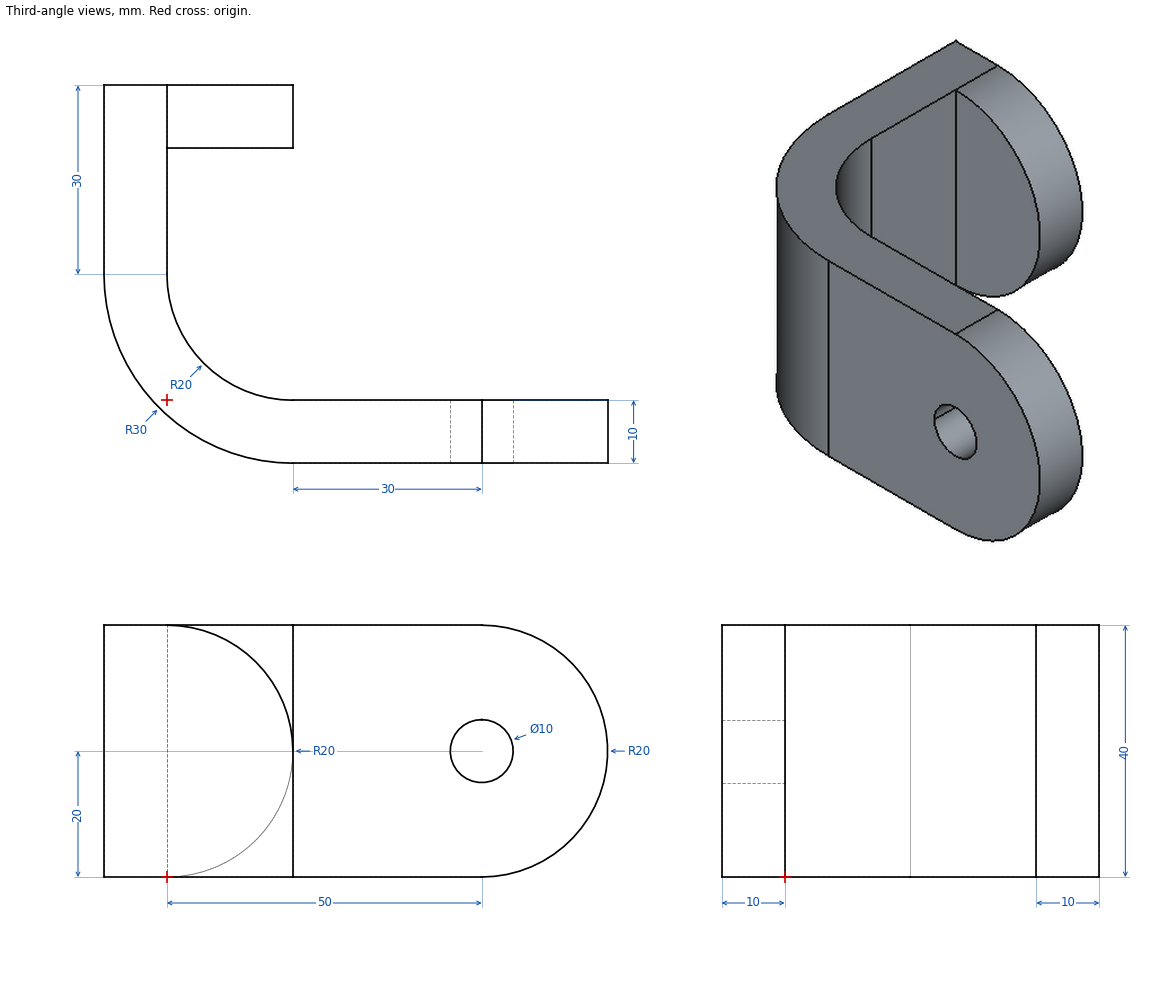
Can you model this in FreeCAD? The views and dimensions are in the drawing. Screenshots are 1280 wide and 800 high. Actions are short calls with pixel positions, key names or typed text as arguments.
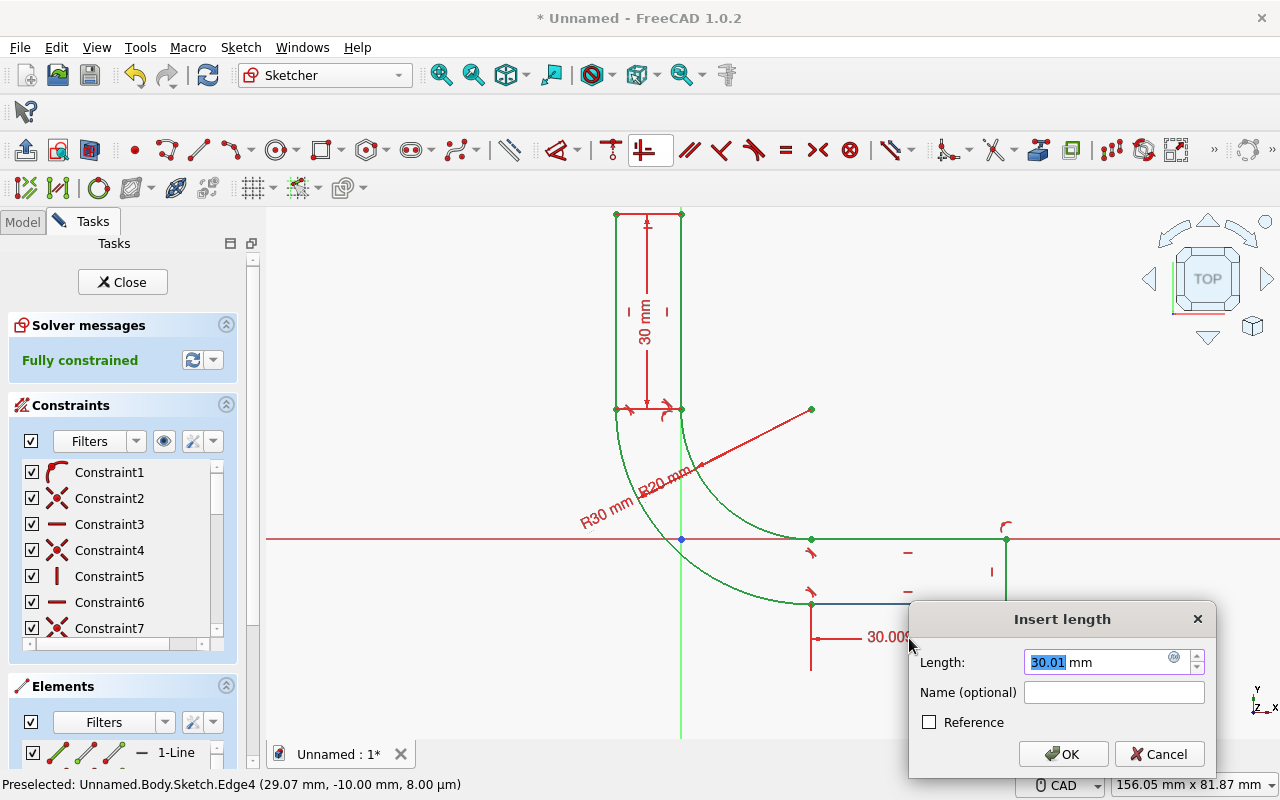
text(30)
key(Return)
key(Escape)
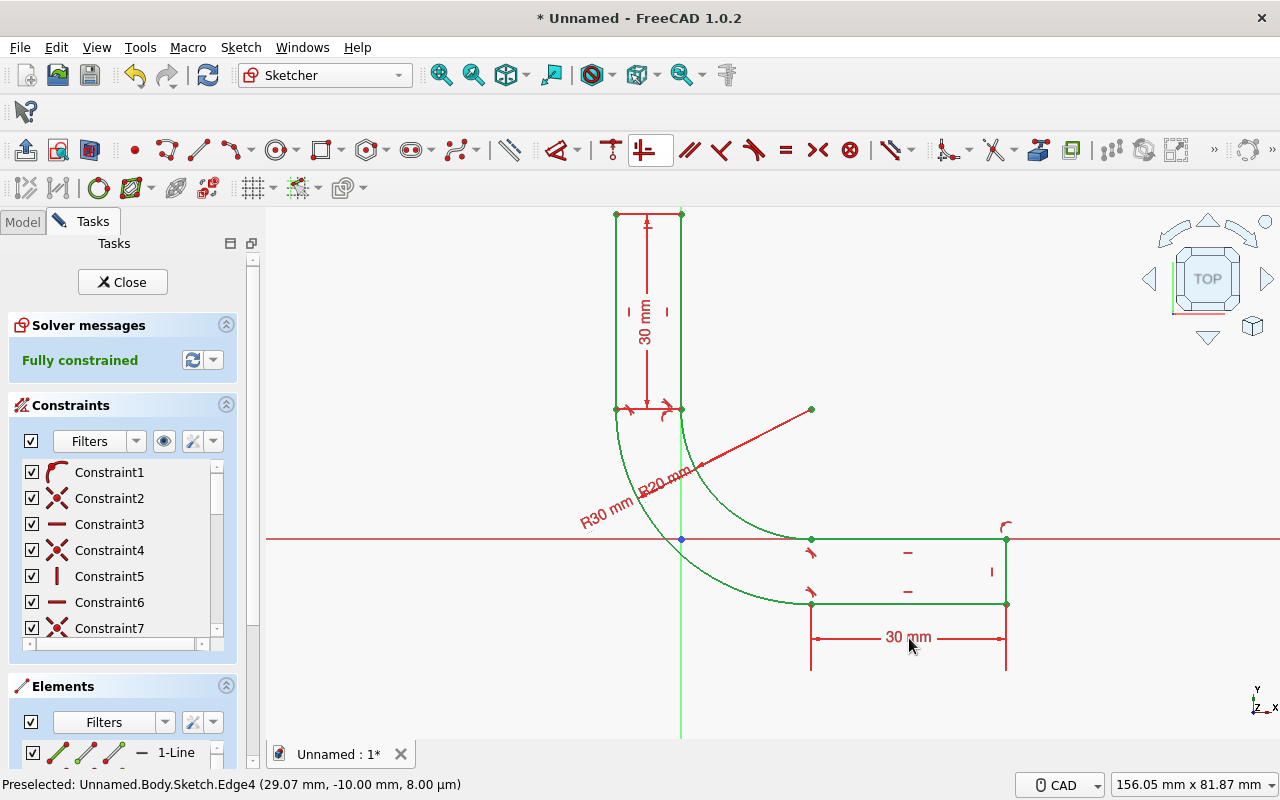
click(123, 282)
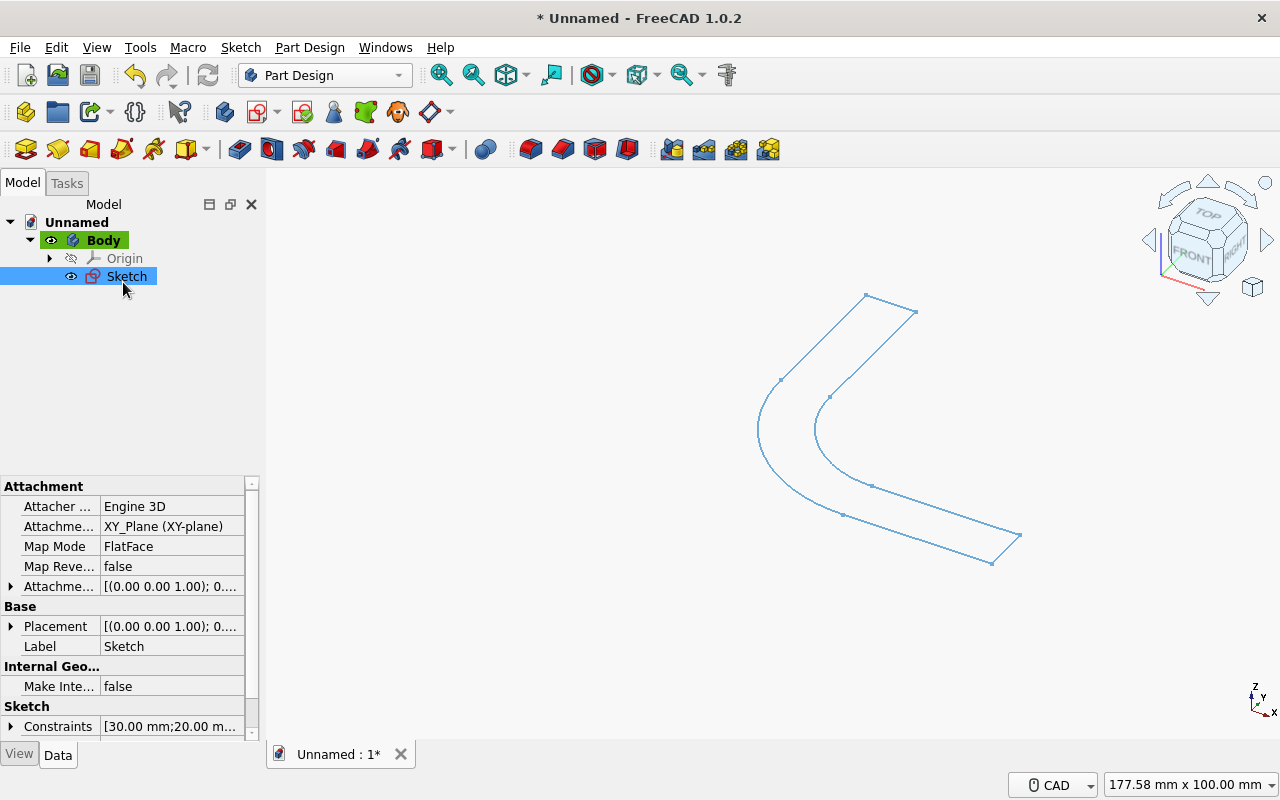
click(26, 150)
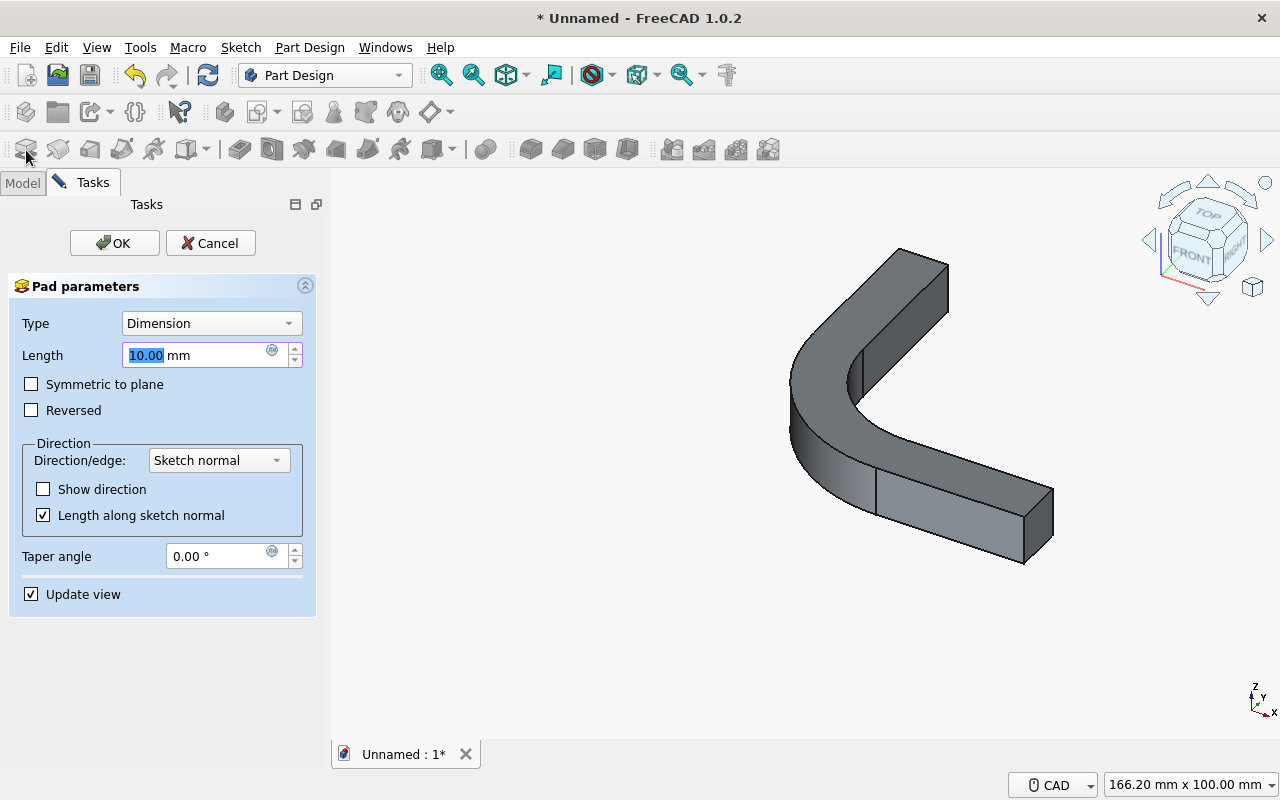
text(40)
key(Tab)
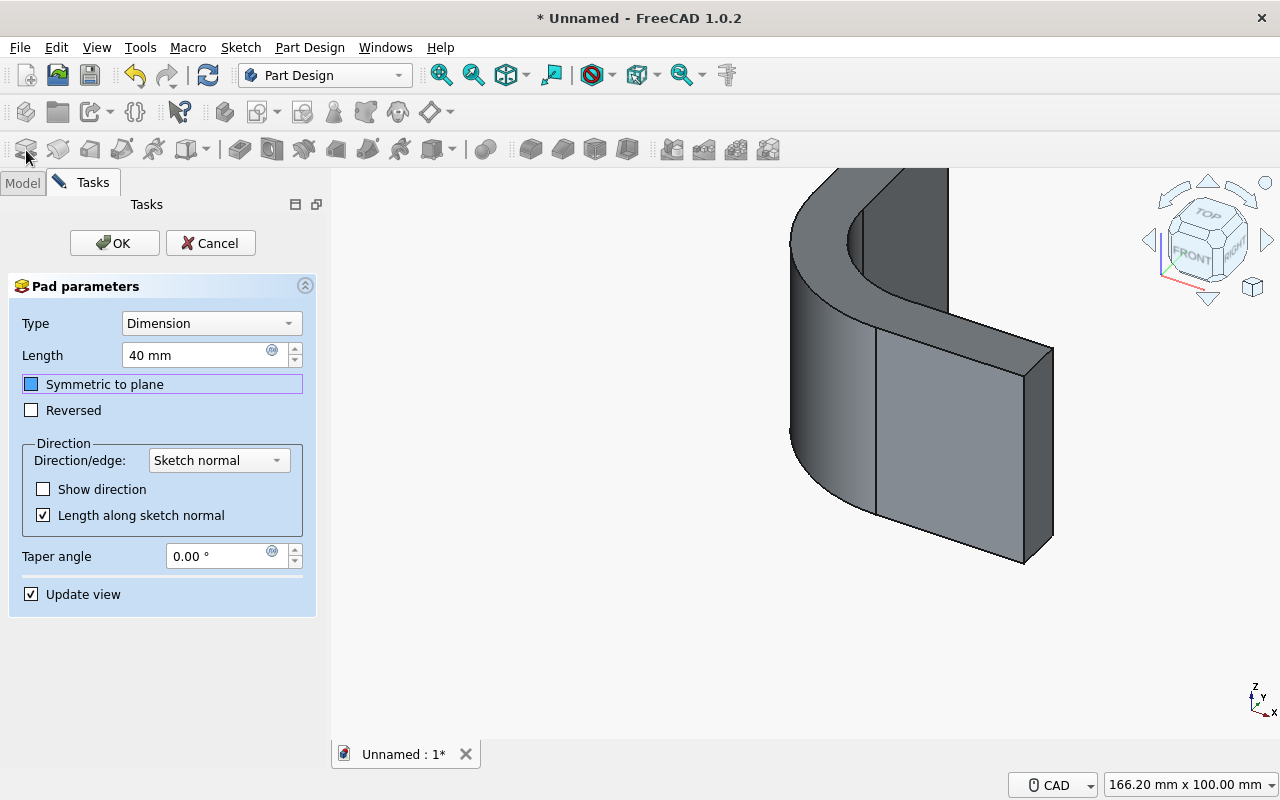
click(115, 243)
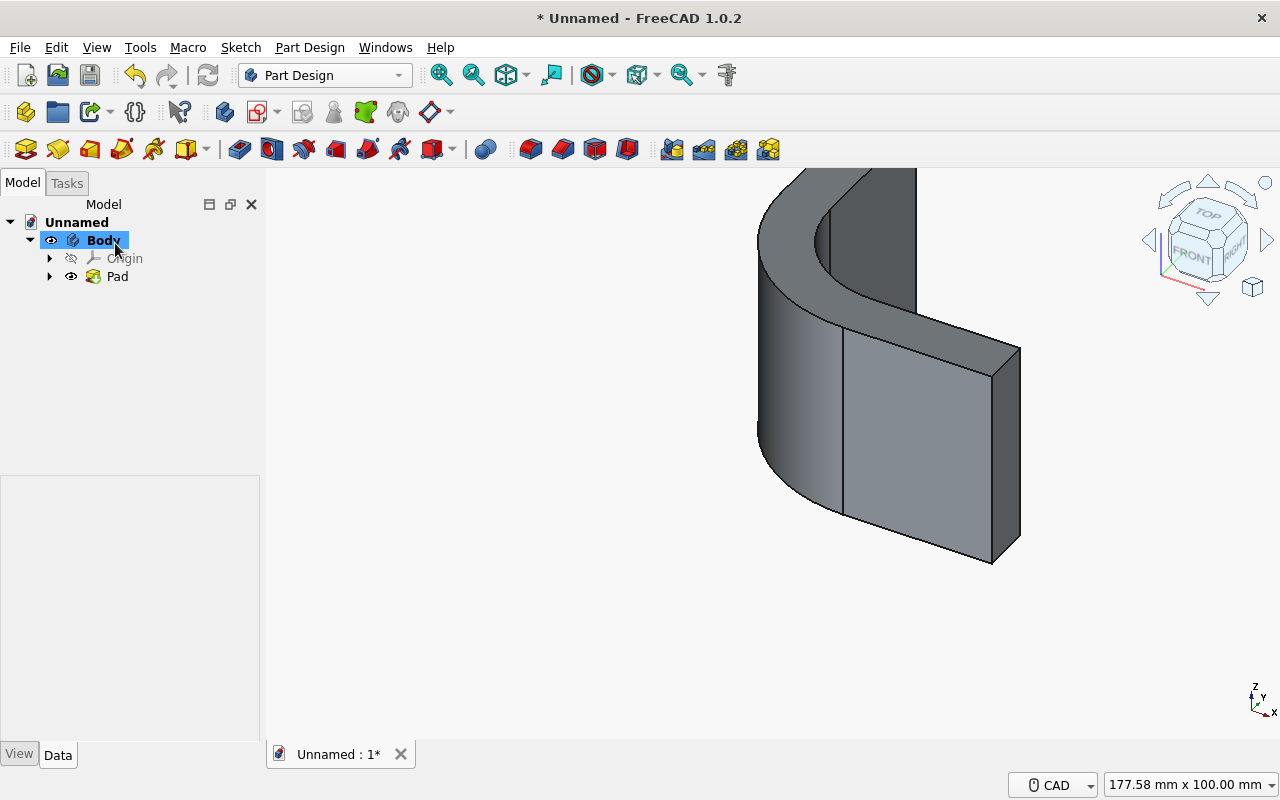
key(v)
key(f)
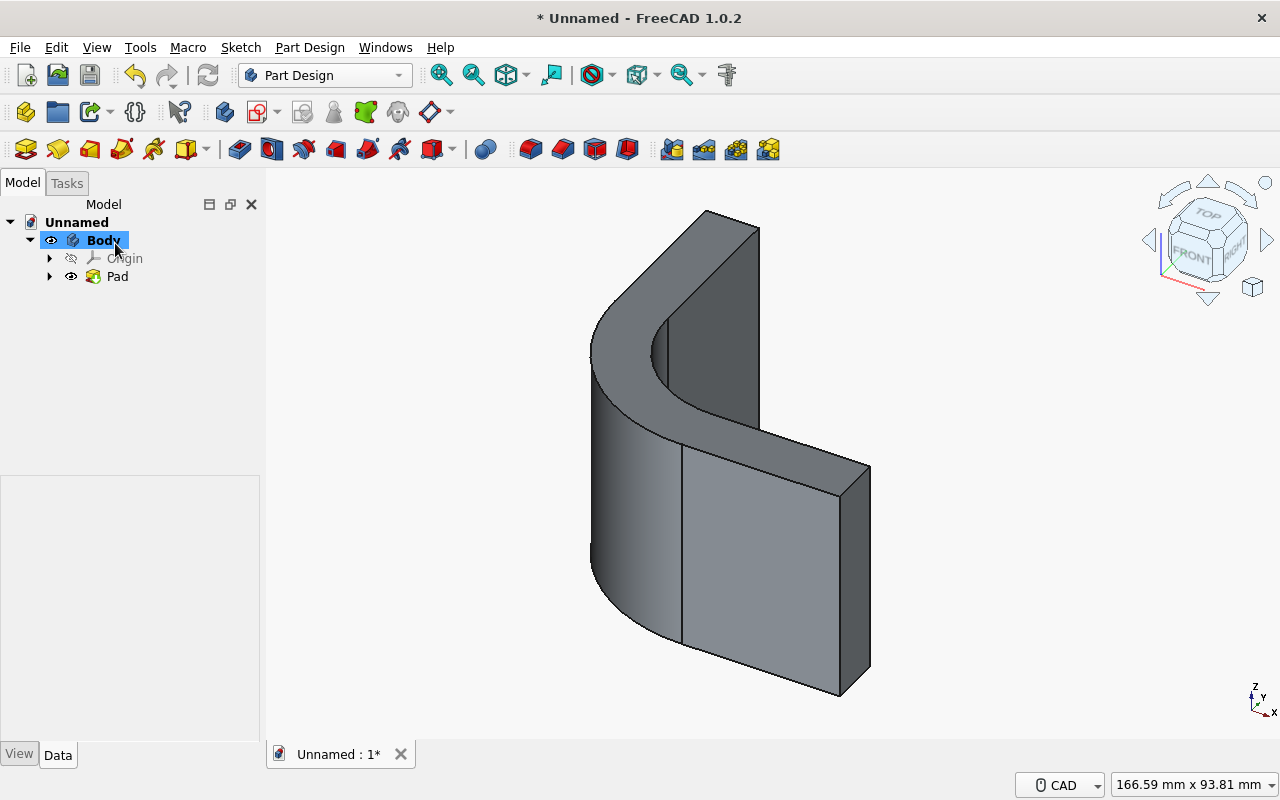
key(4)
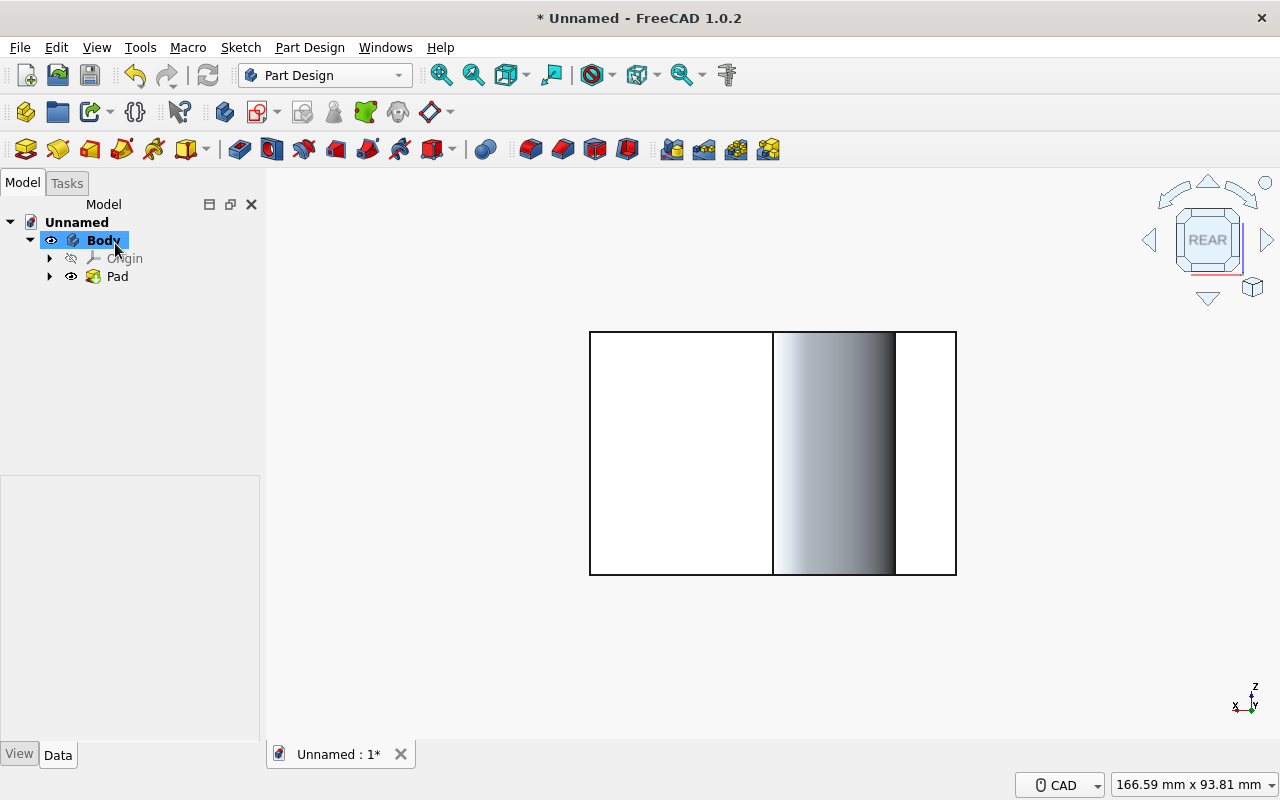
key(v)
key(f)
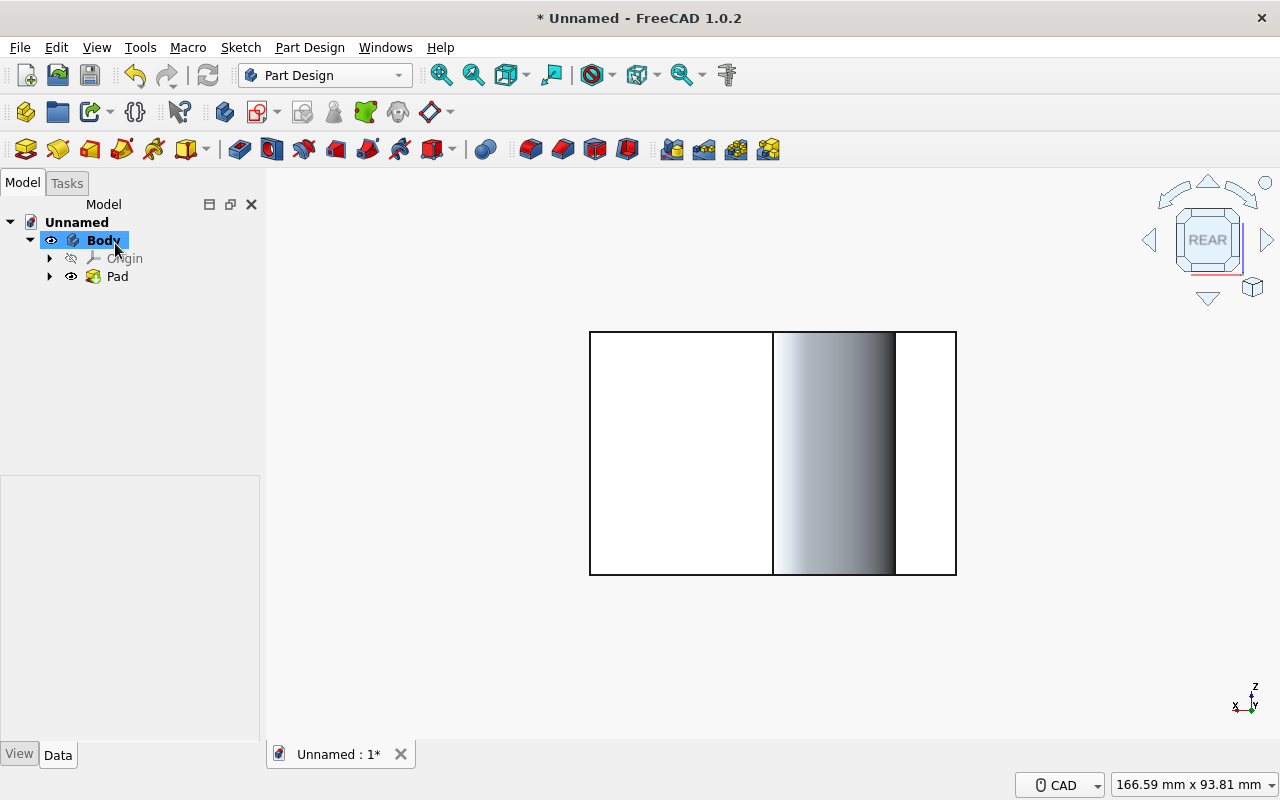
click(925, 383)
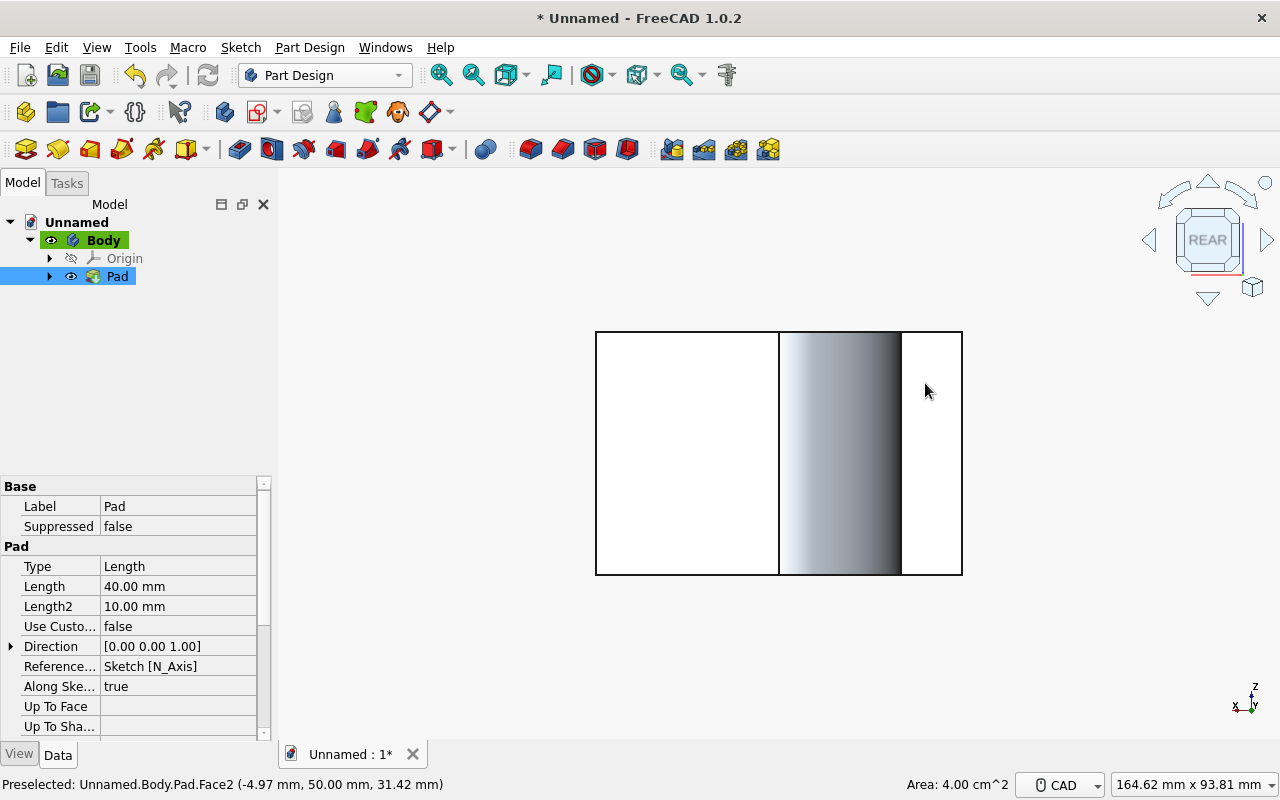
click(258, 112)